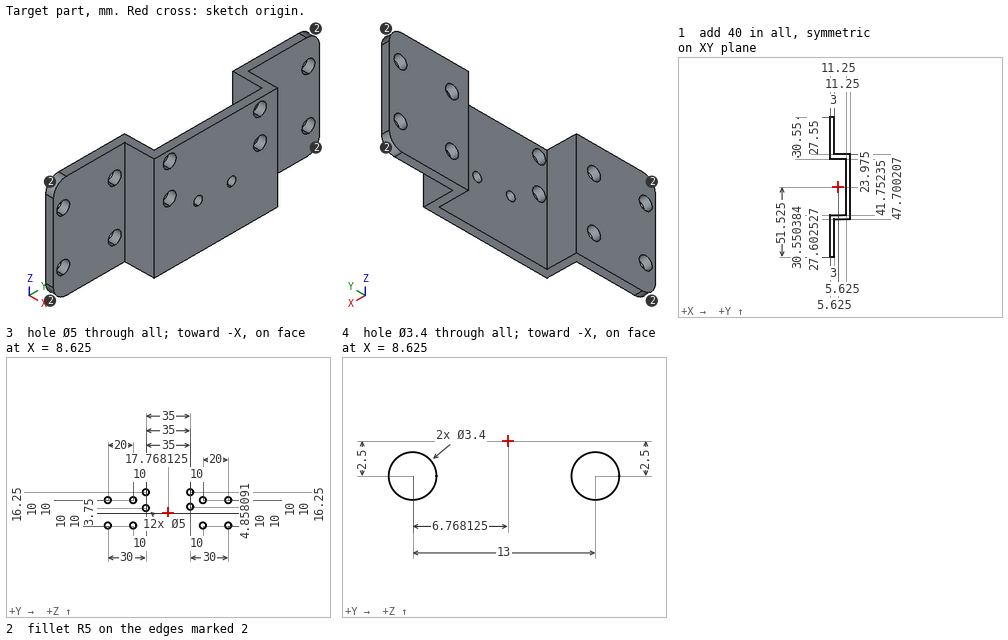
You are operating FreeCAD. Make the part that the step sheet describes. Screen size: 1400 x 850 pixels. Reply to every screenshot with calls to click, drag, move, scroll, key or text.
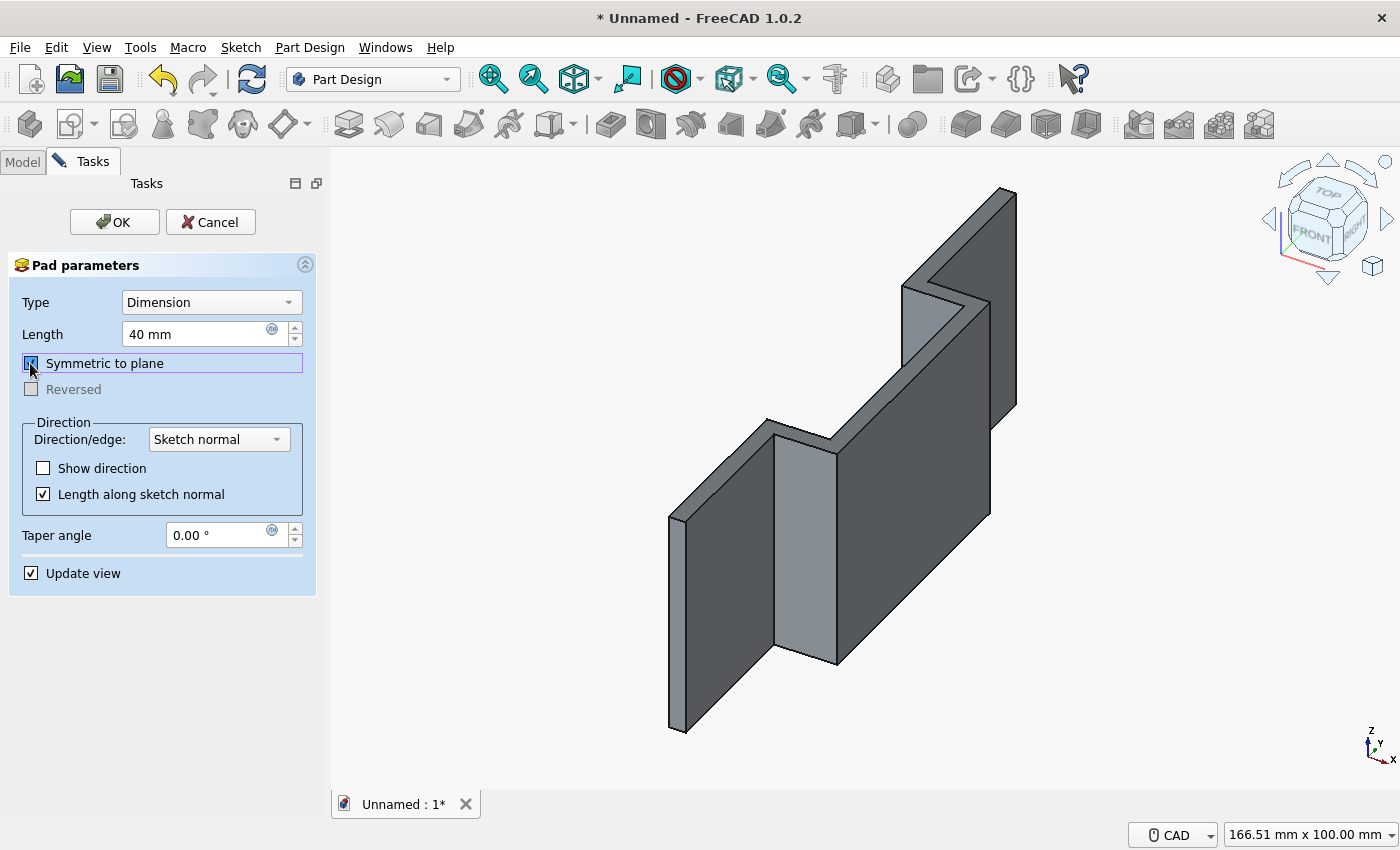
click(115, 222)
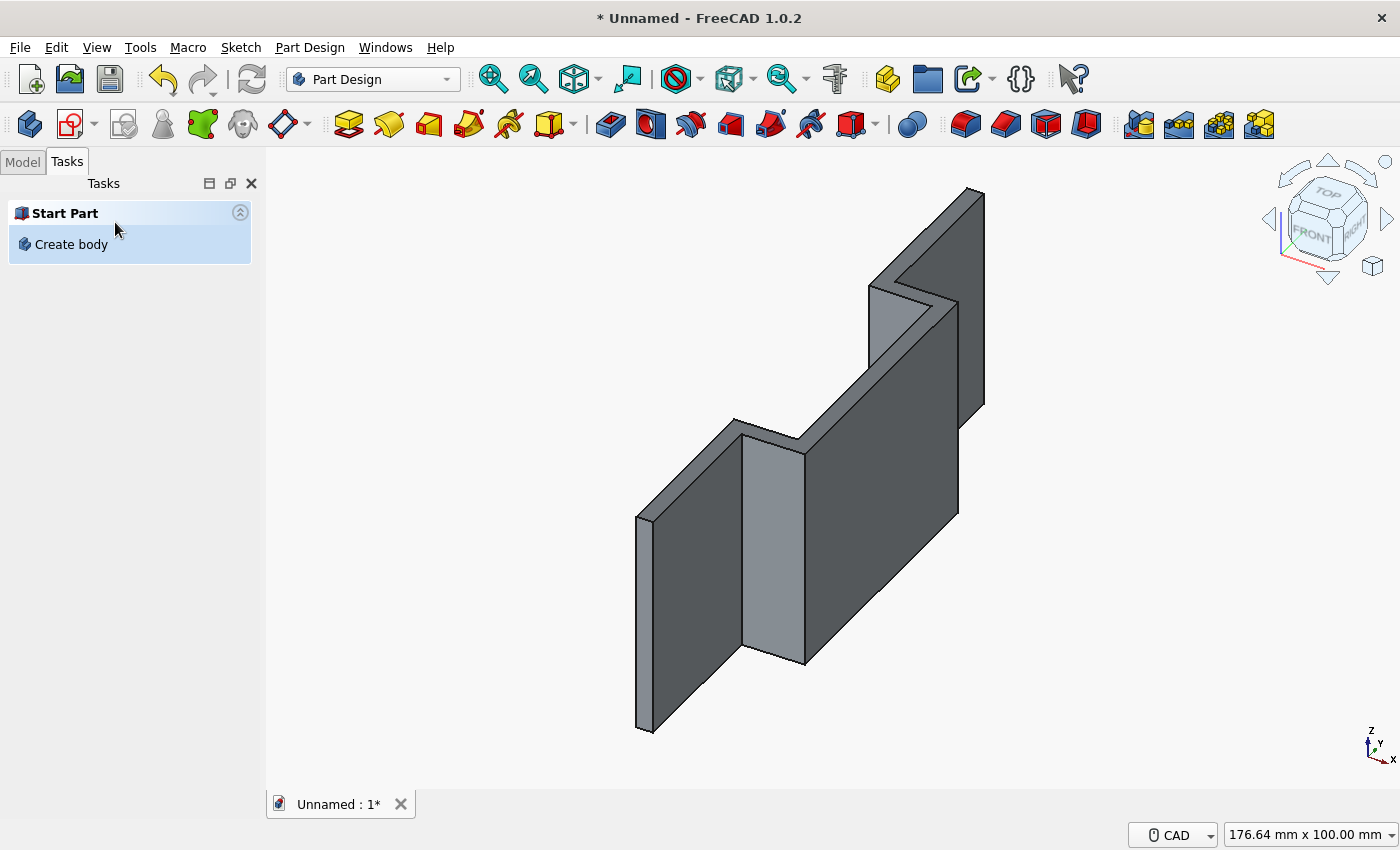
click(645, 519)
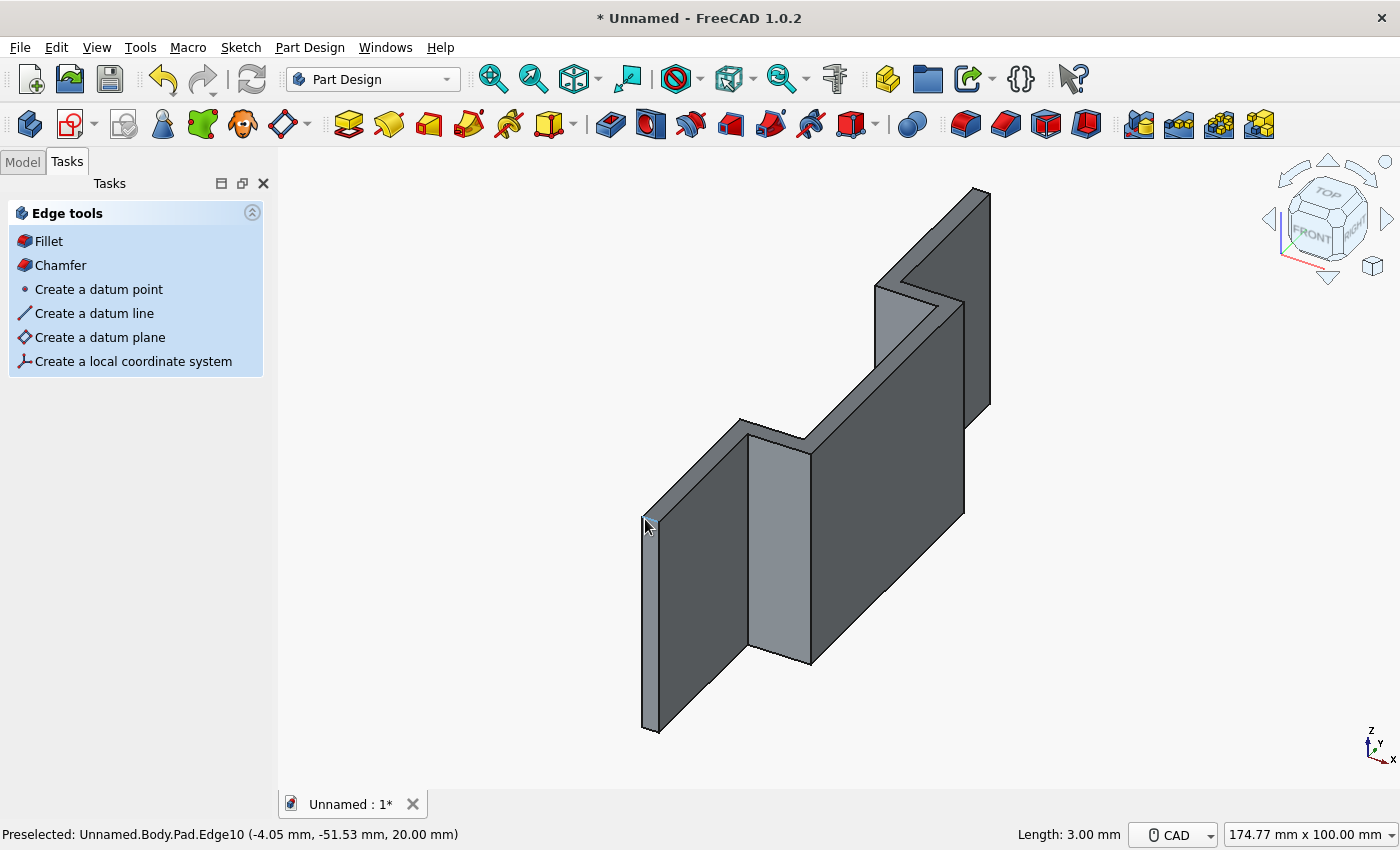
scroll(981, 400, up, 4)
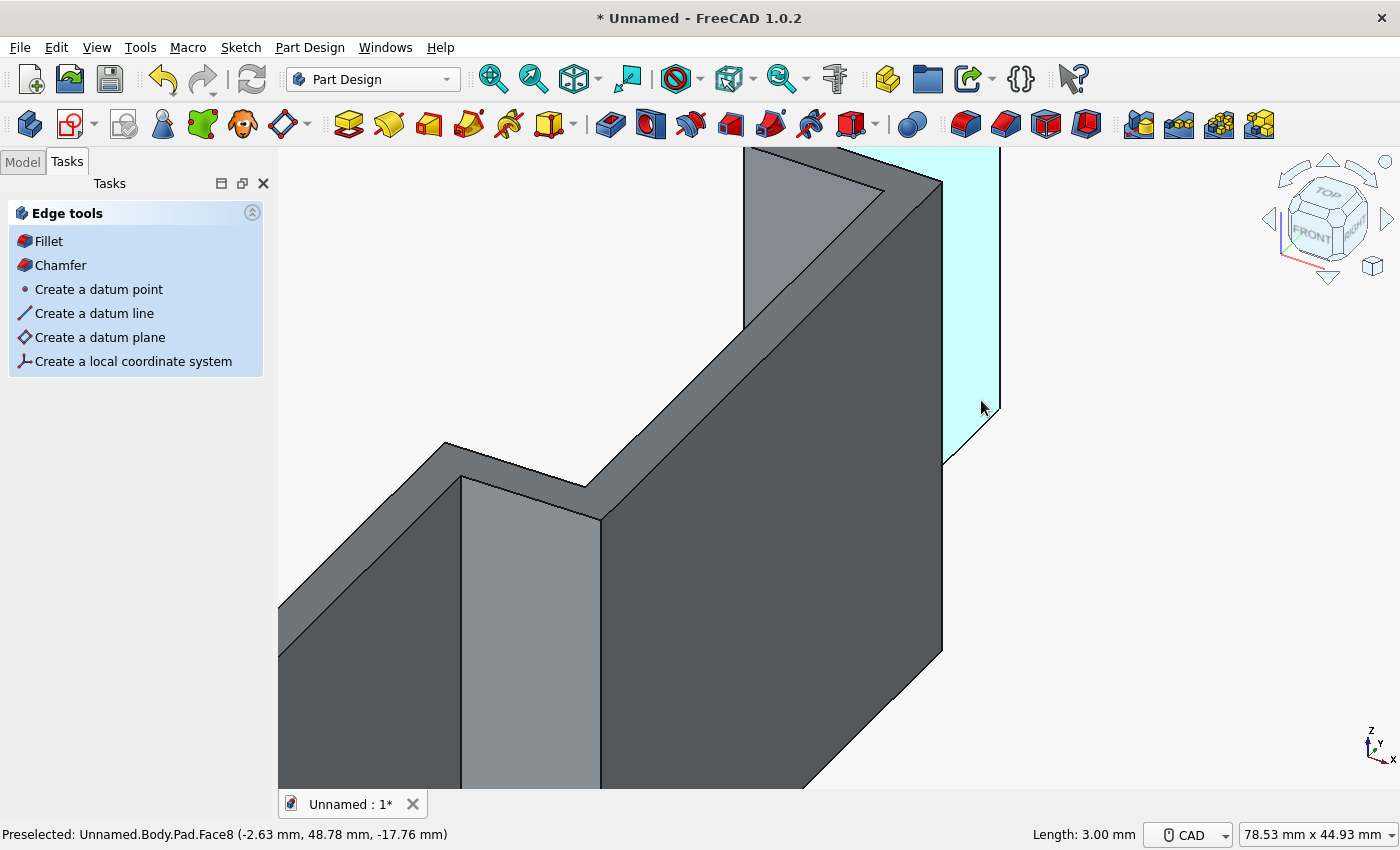
click(494, 80)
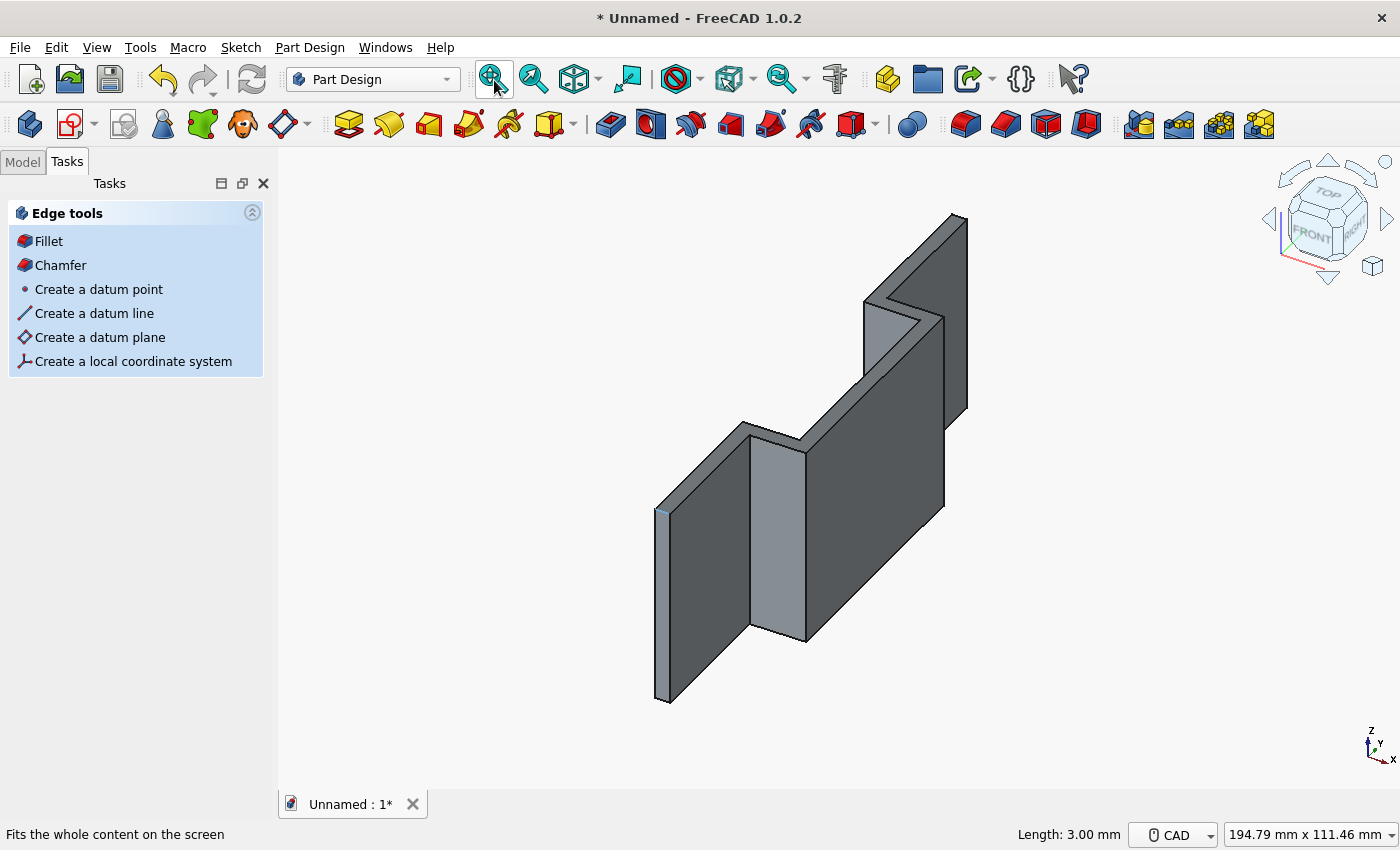
key(0)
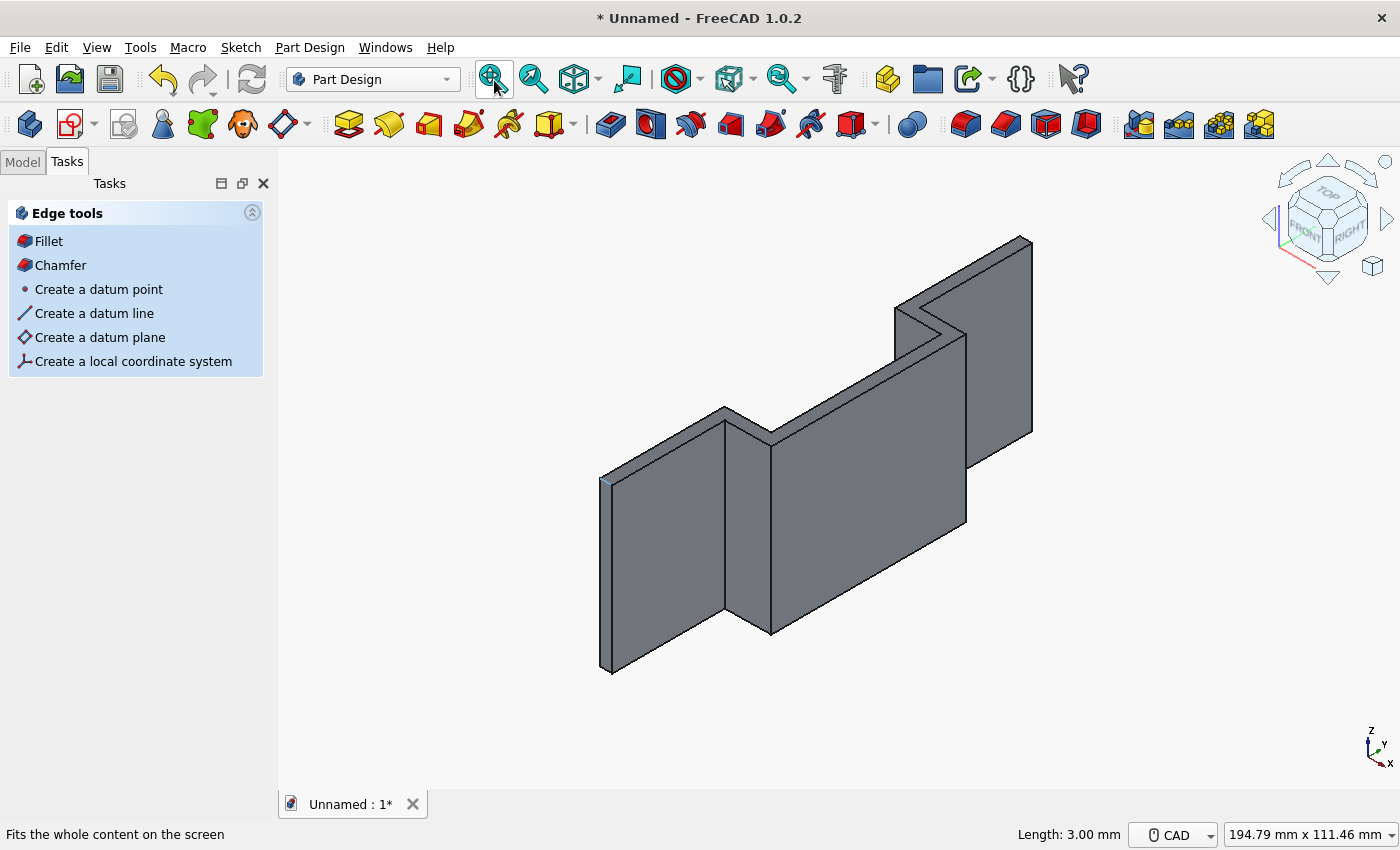
scroll(1026, 427, up, 5)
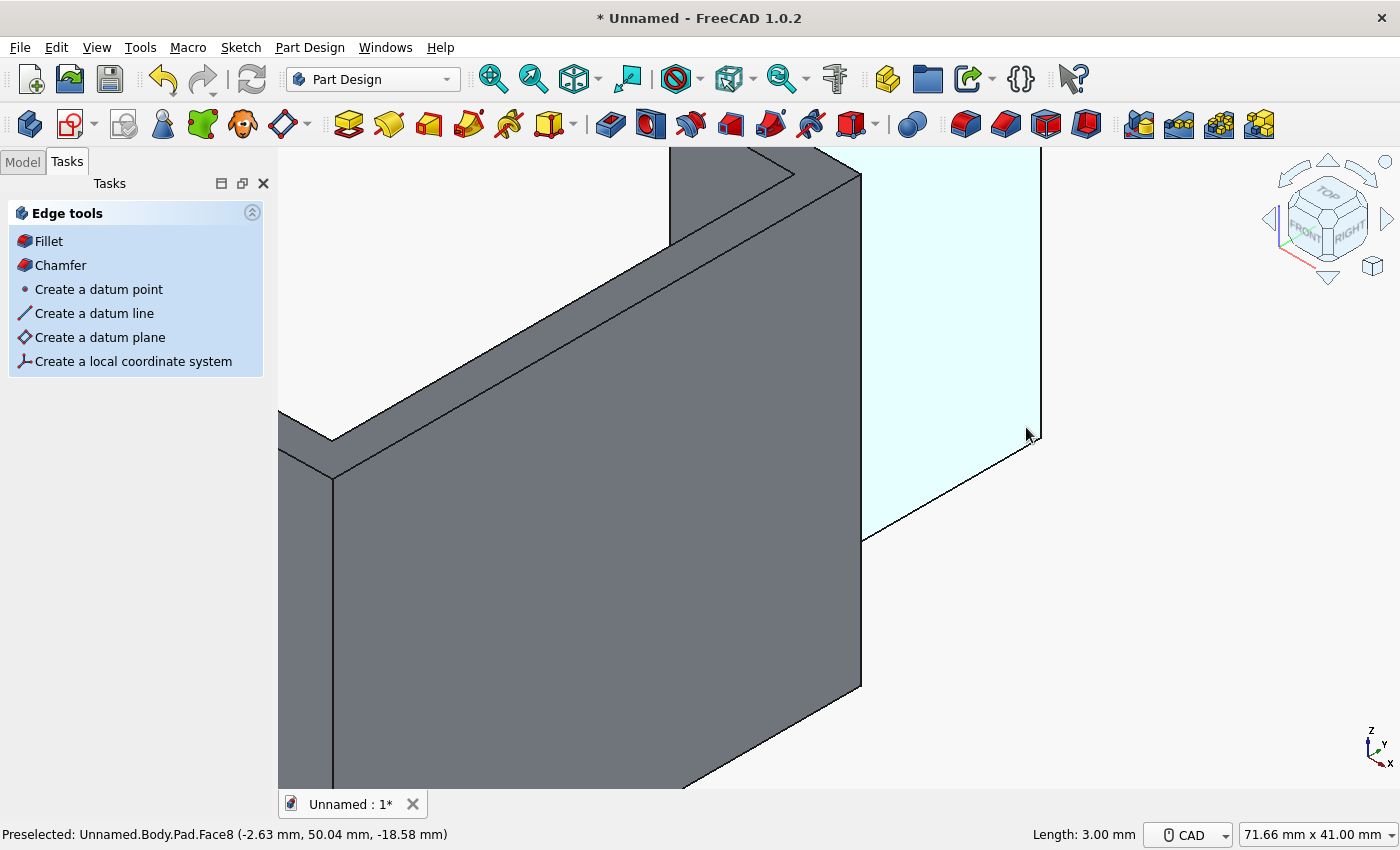
key(v)
key(f)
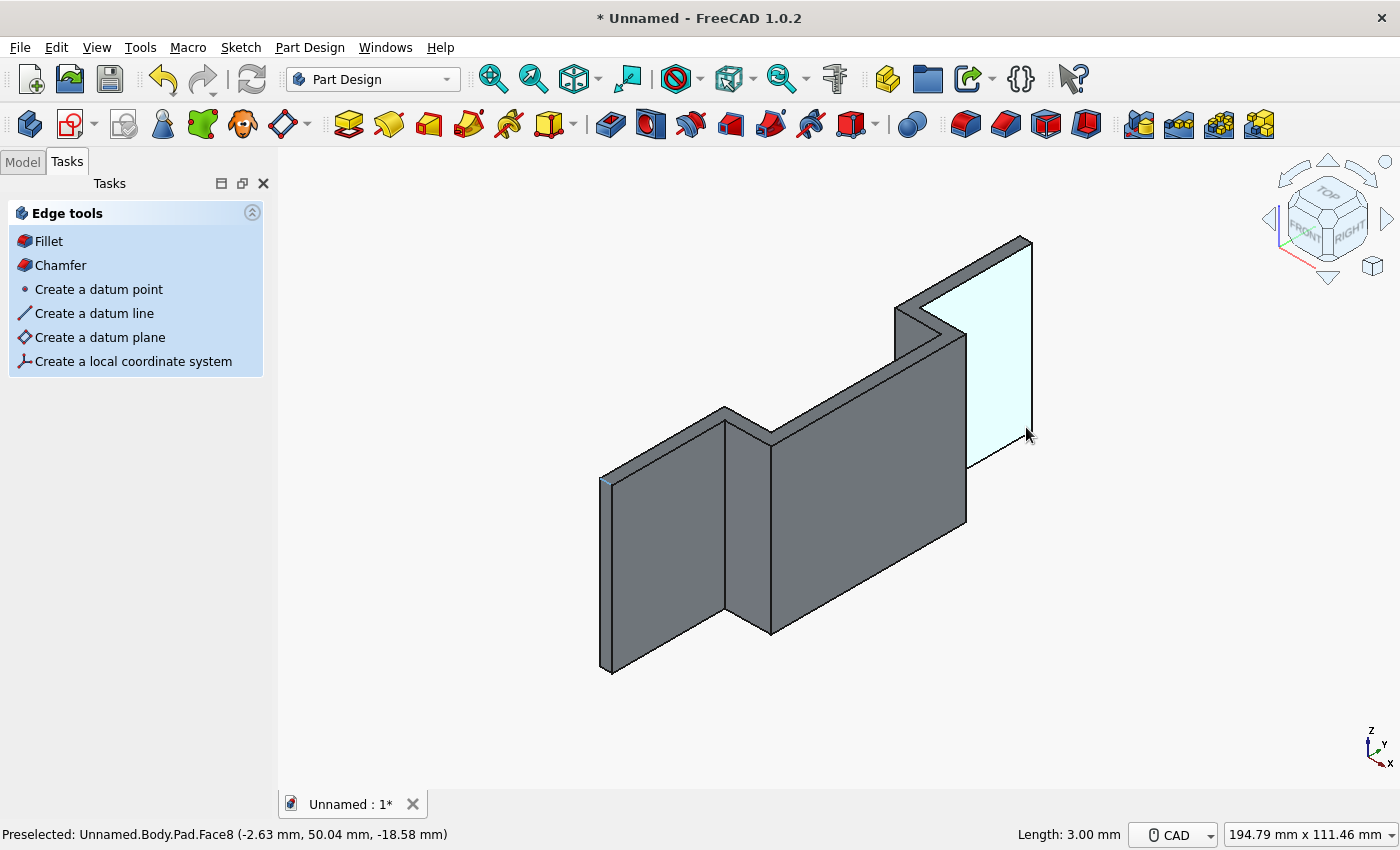
key(2)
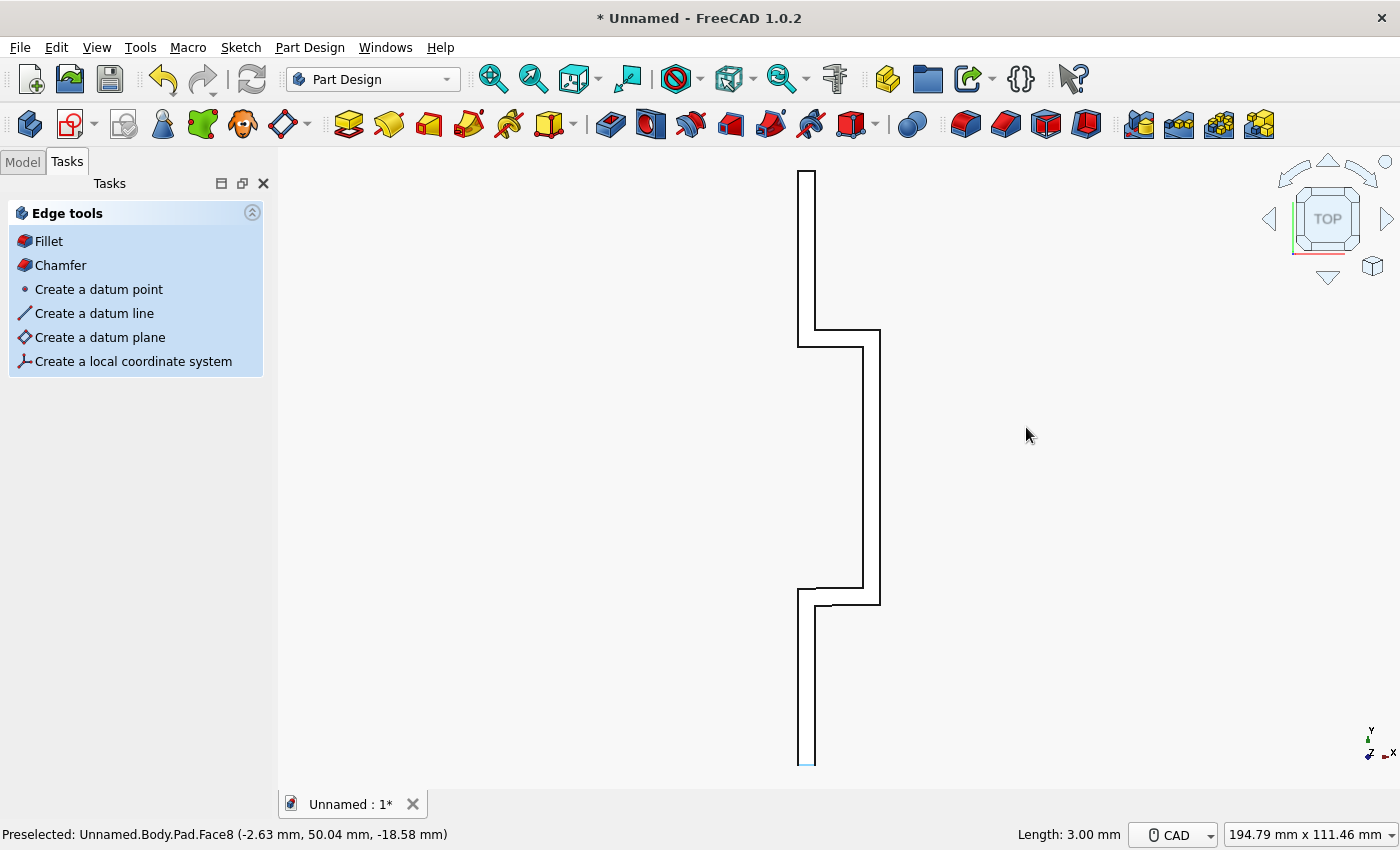
key(1)